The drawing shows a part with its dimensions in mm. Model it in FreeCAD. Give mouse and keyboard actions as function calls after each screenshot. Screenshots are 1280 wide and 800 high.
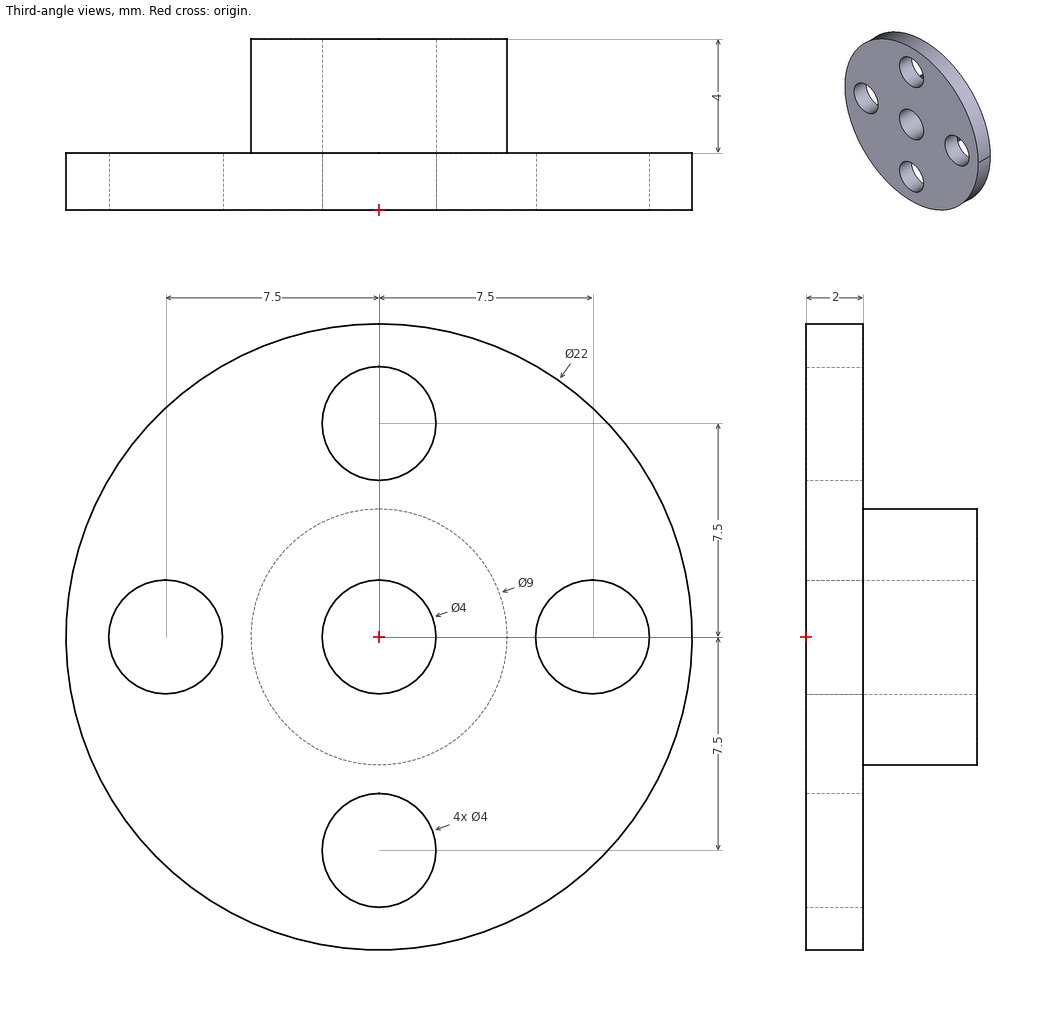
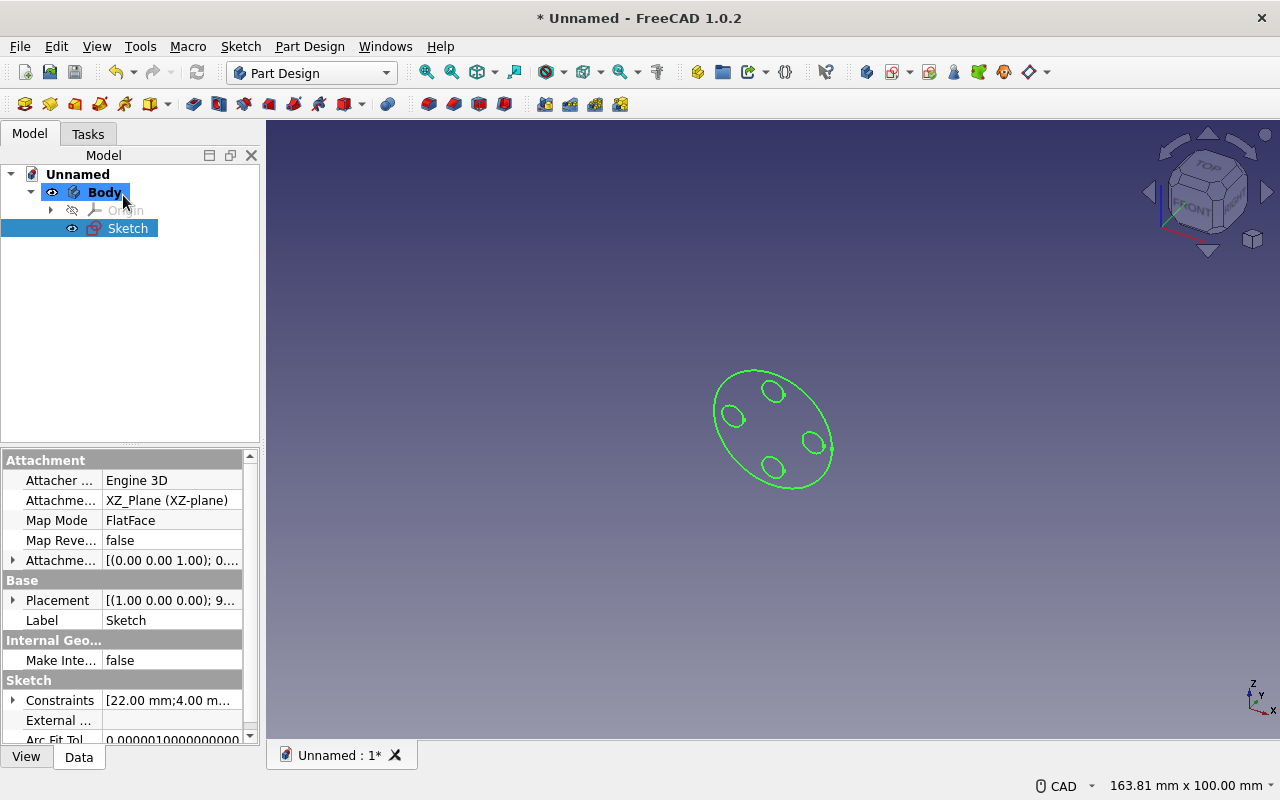
click(25, 104)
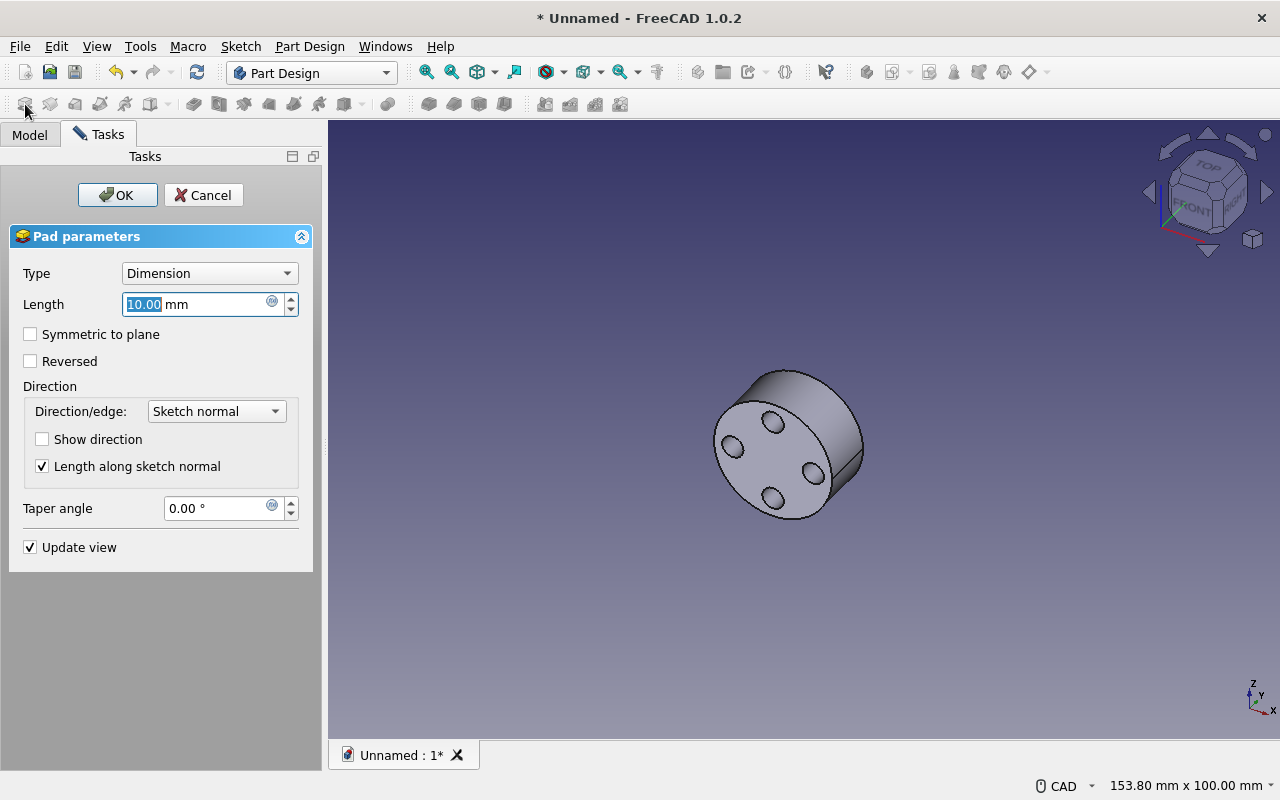
text(2)
key(Tab)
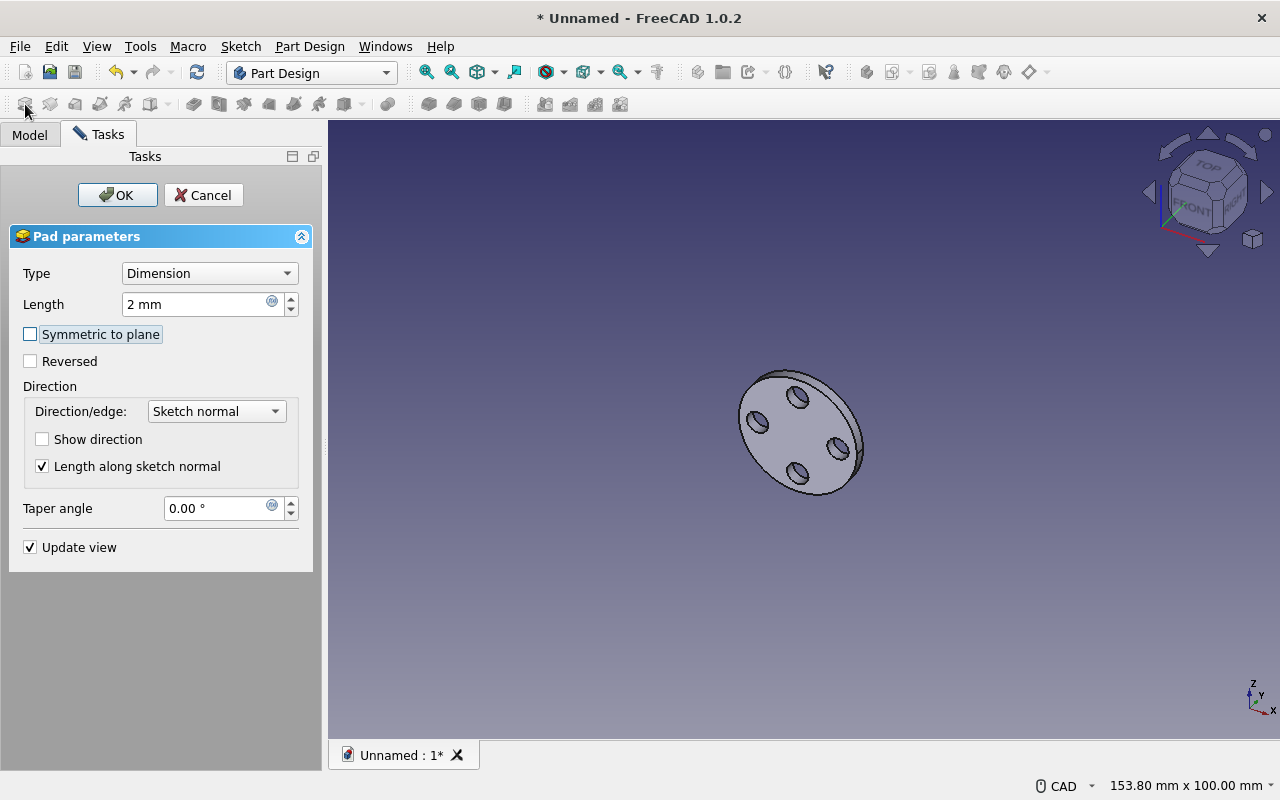
click(31, 361)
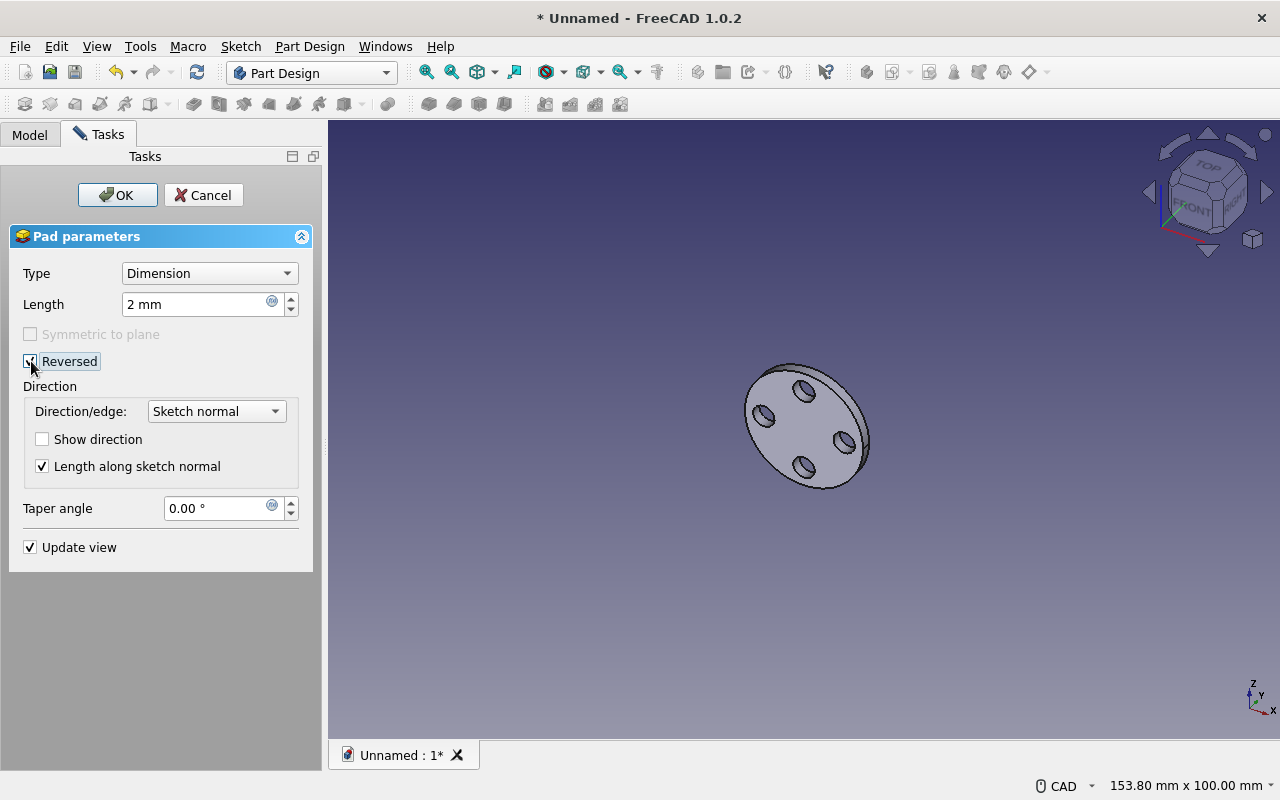
click(118, 195)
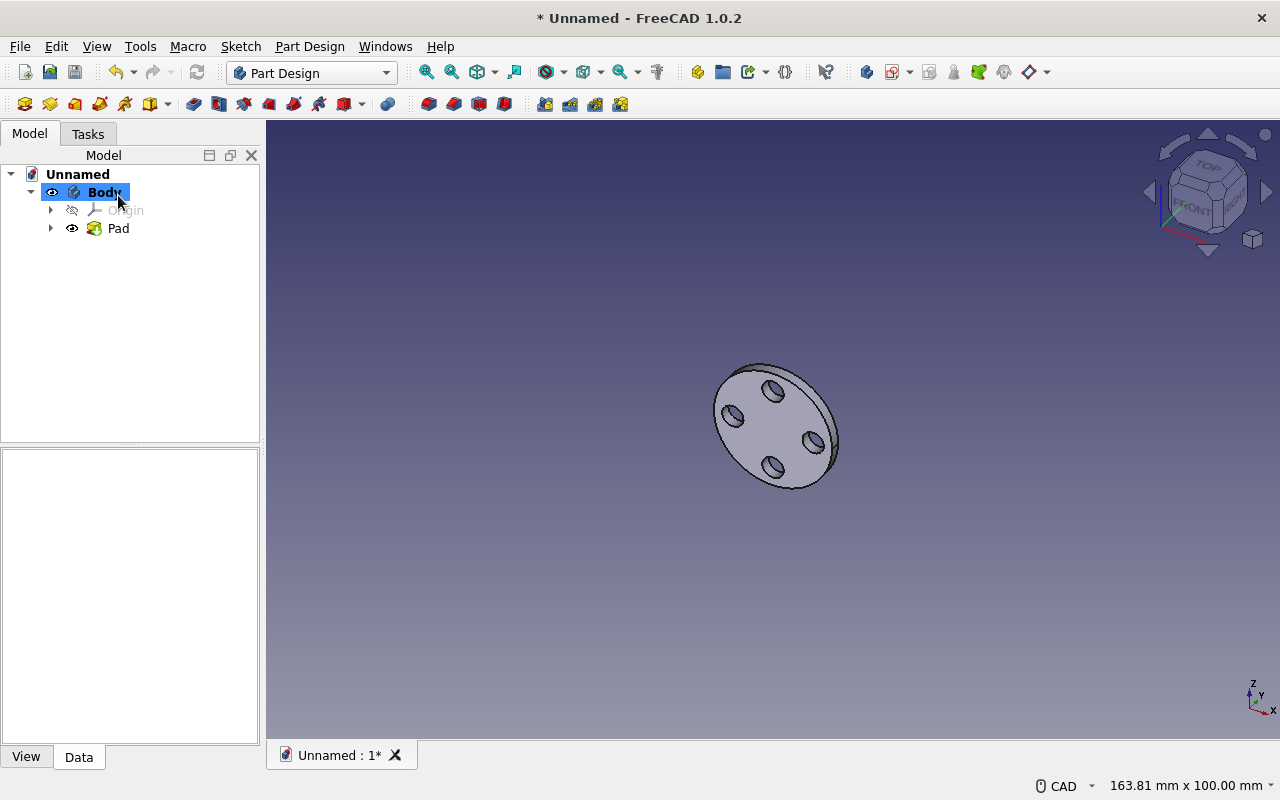
click(427, 72)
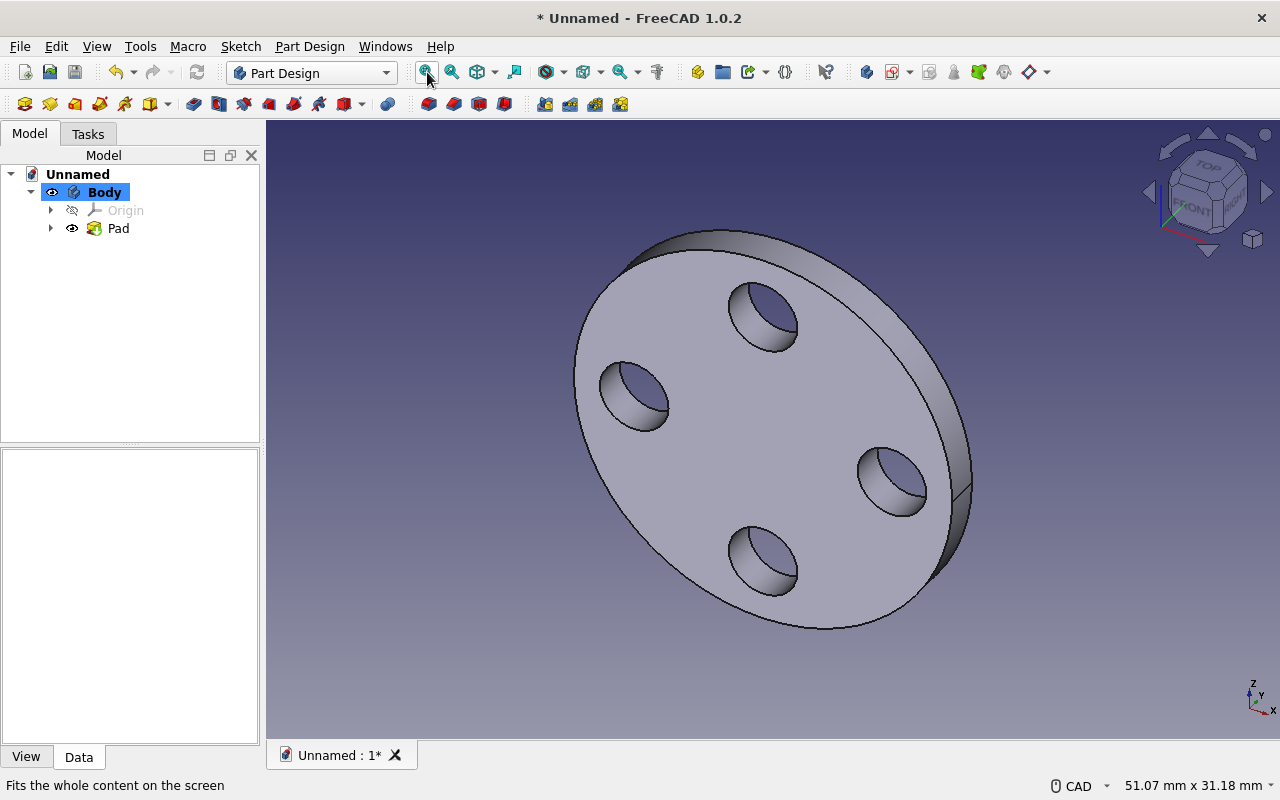
key(4)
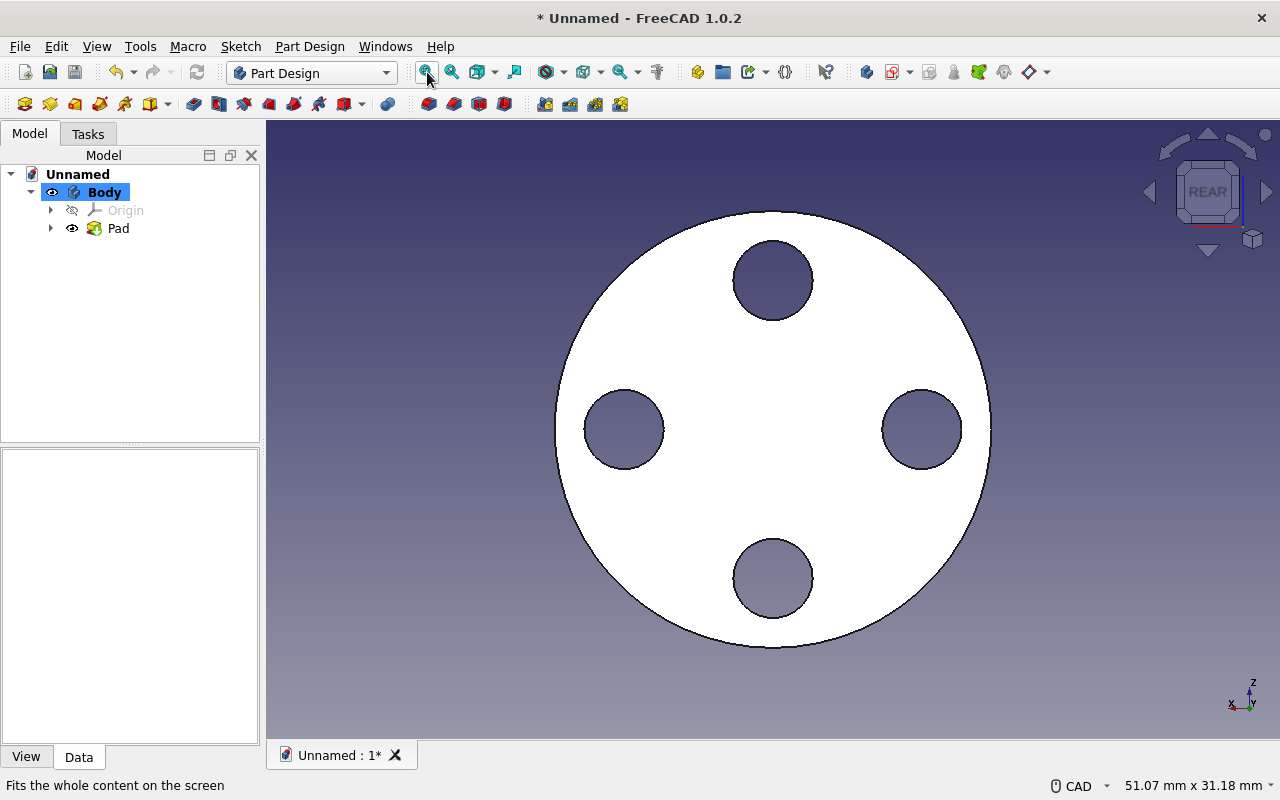
click(773, 429)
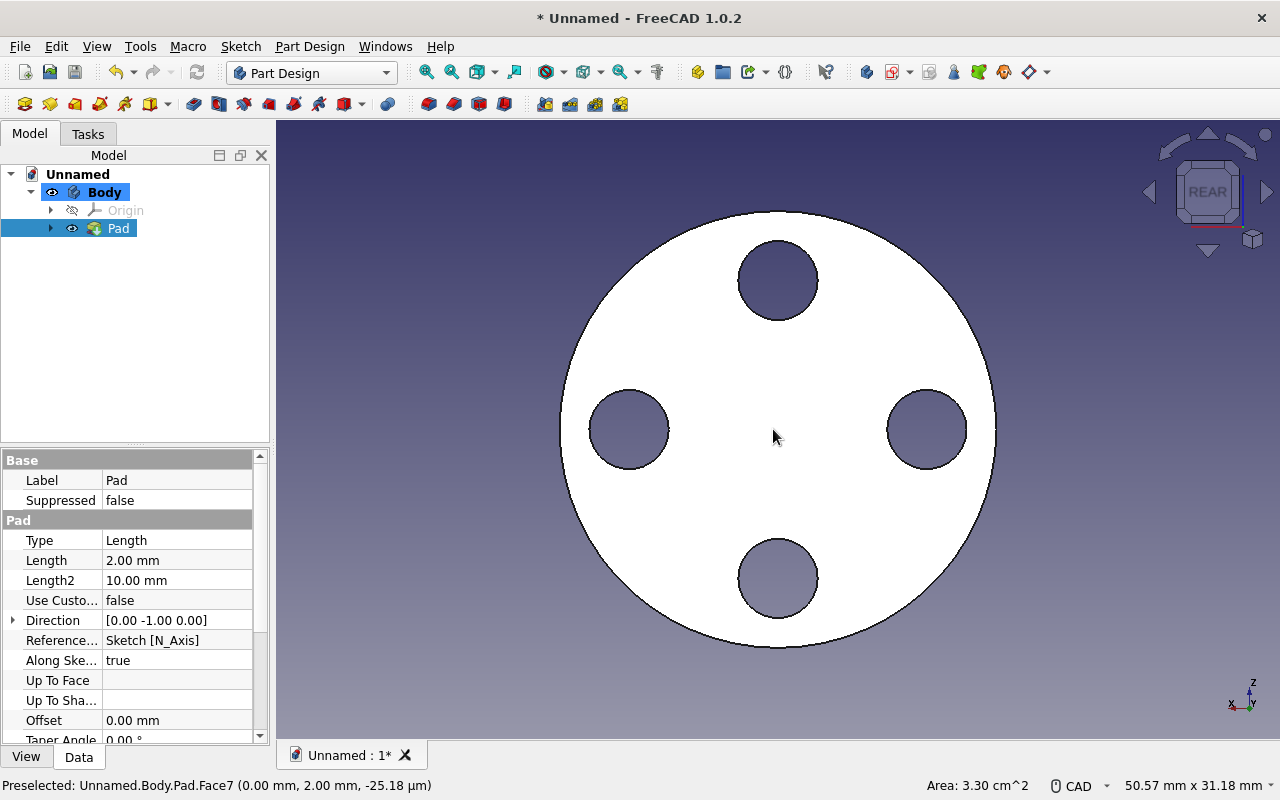
click(892, 72)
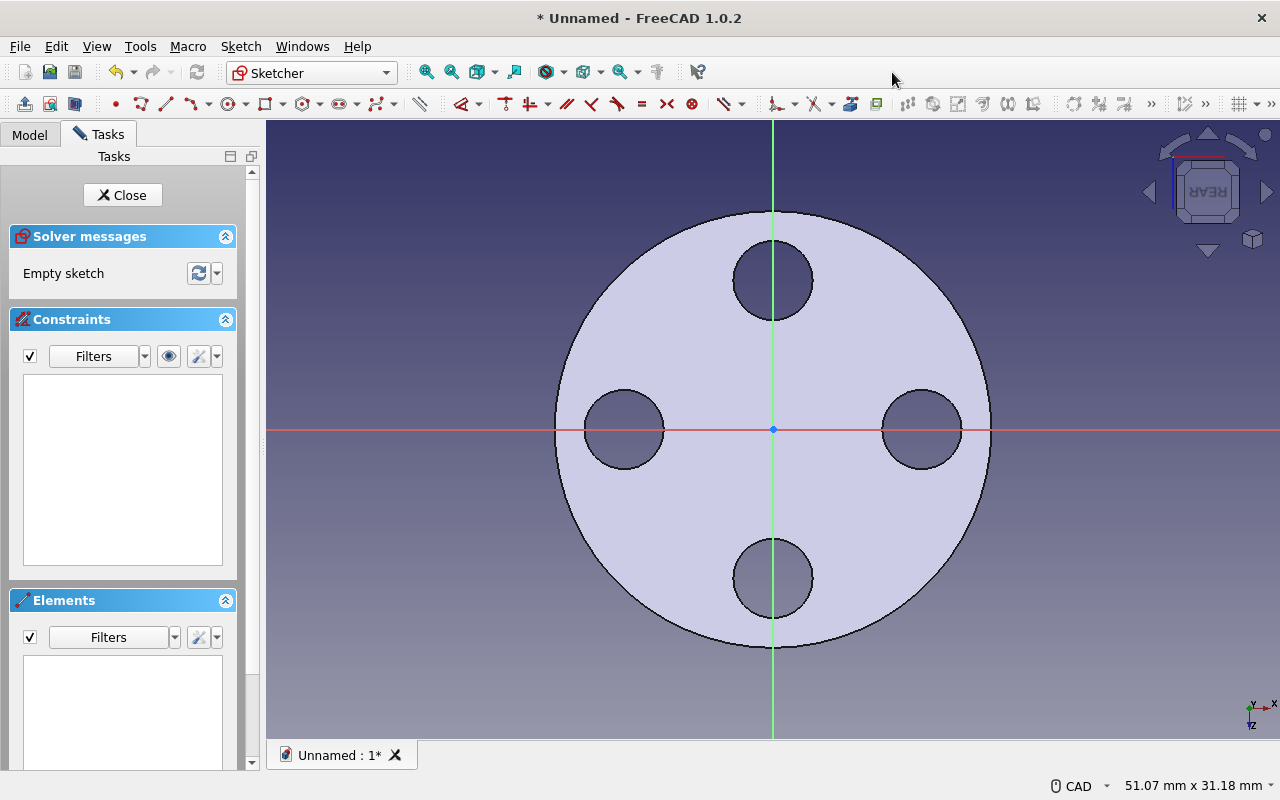
scroll(829, 429, up, 4)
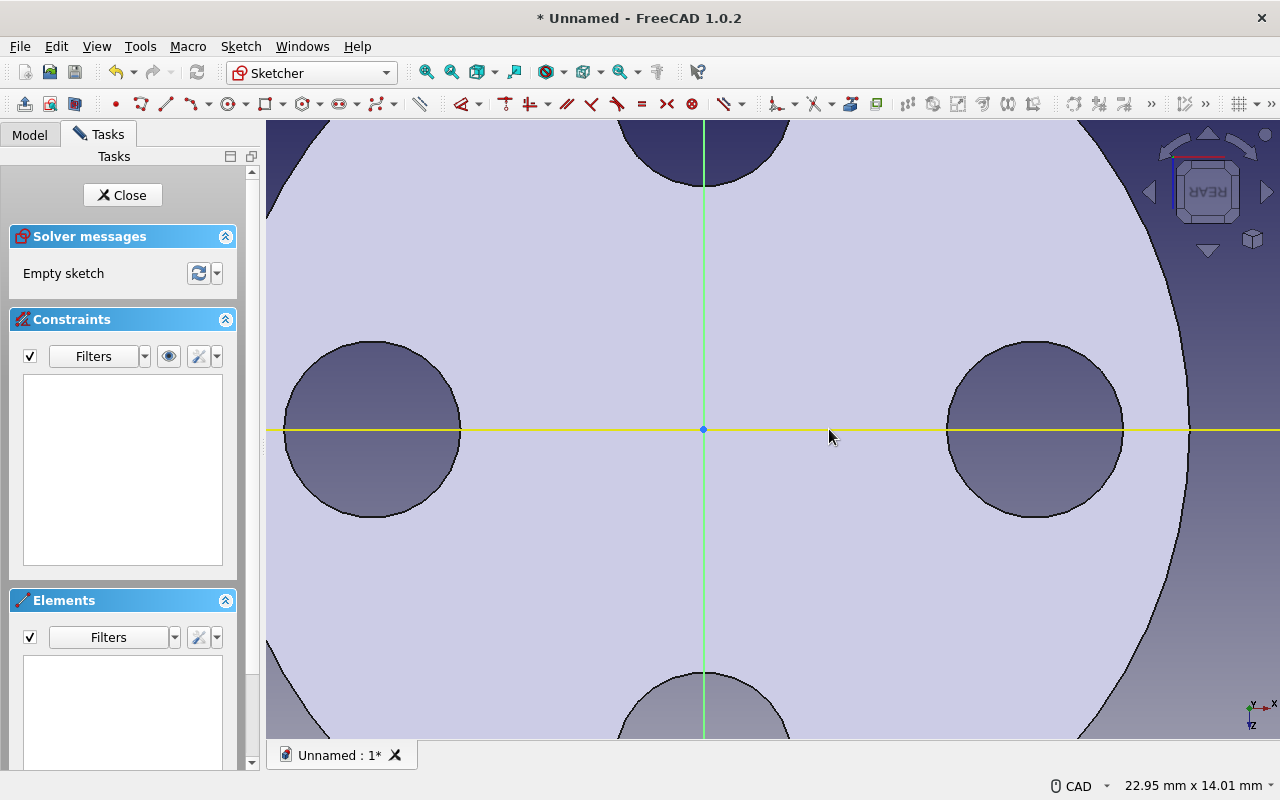
click(228, 104)